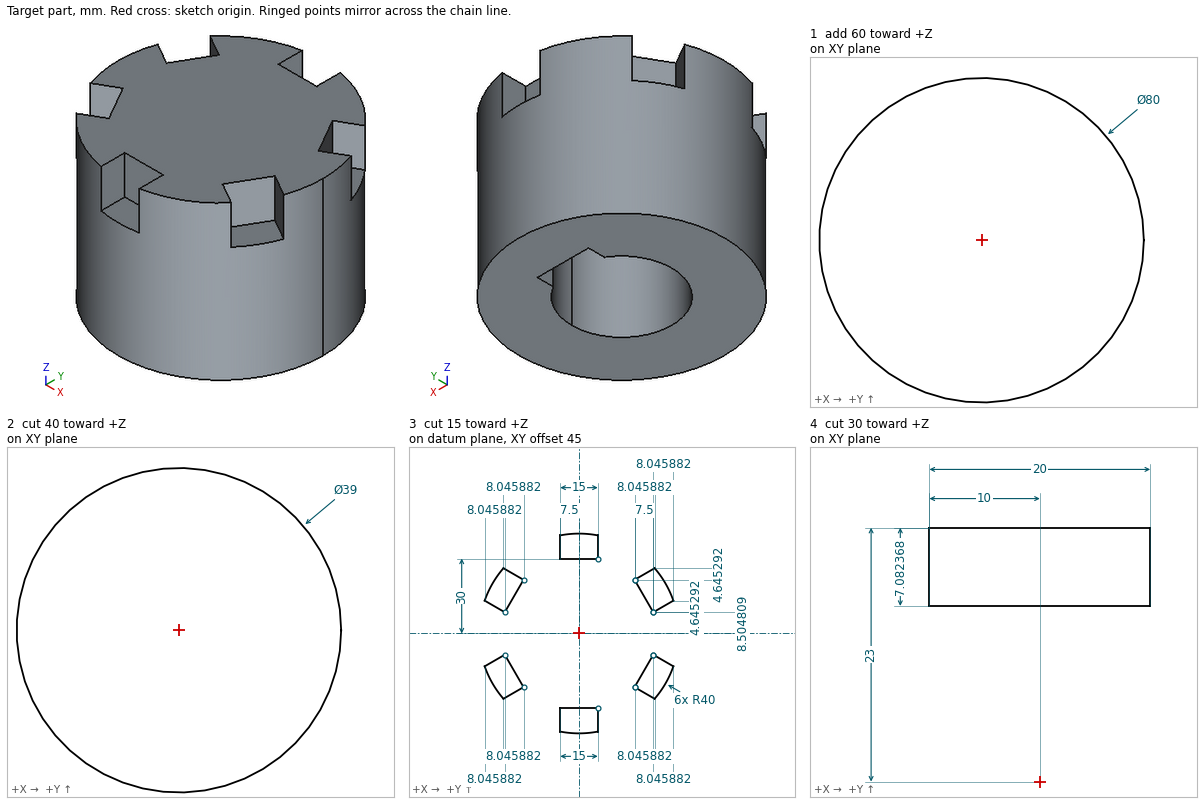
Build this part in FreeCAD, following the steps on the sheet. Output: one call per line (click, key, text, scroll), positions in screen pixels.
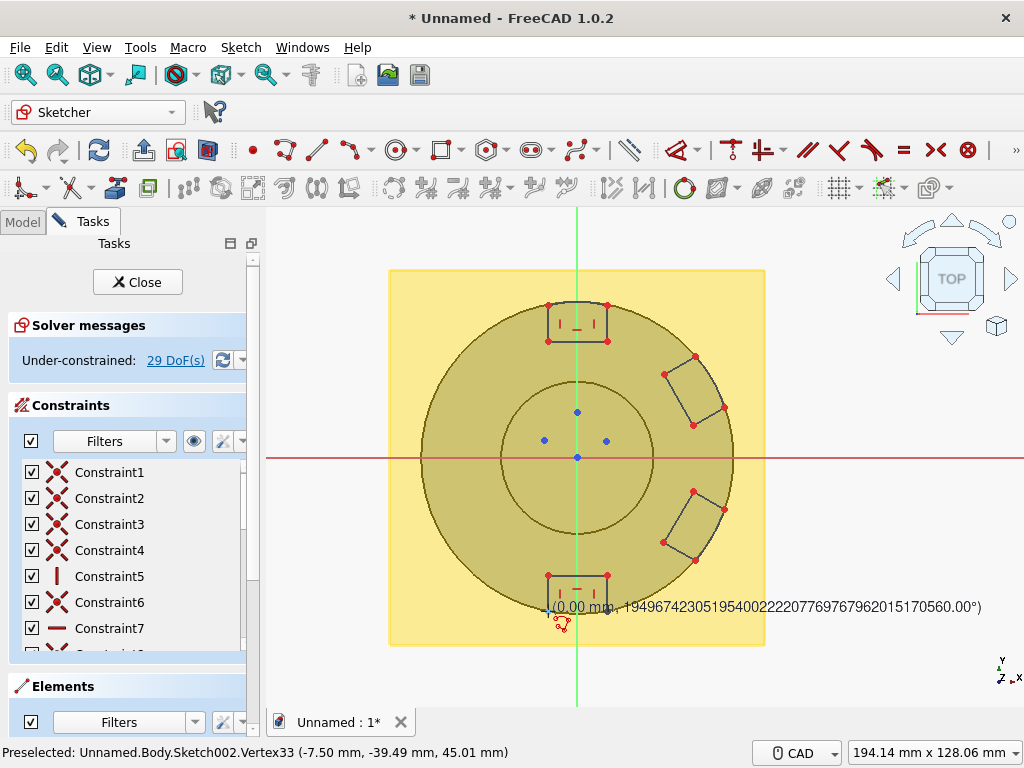
key(g)
key(3)
key(a)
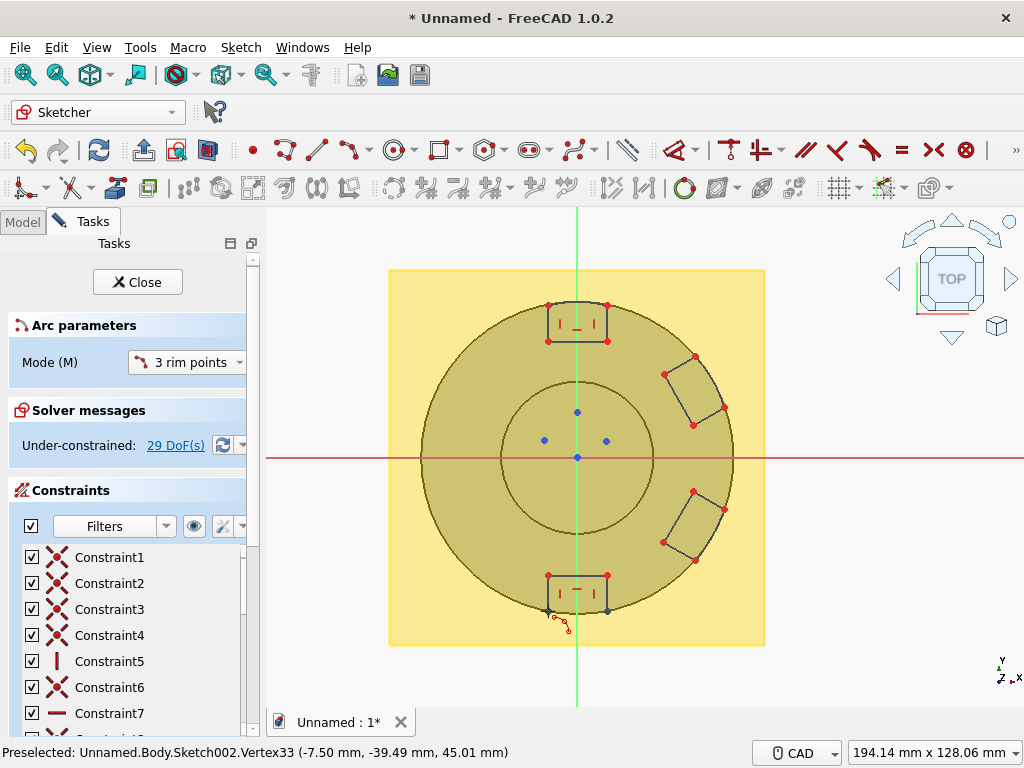
click(548, 612)
click(607, 612)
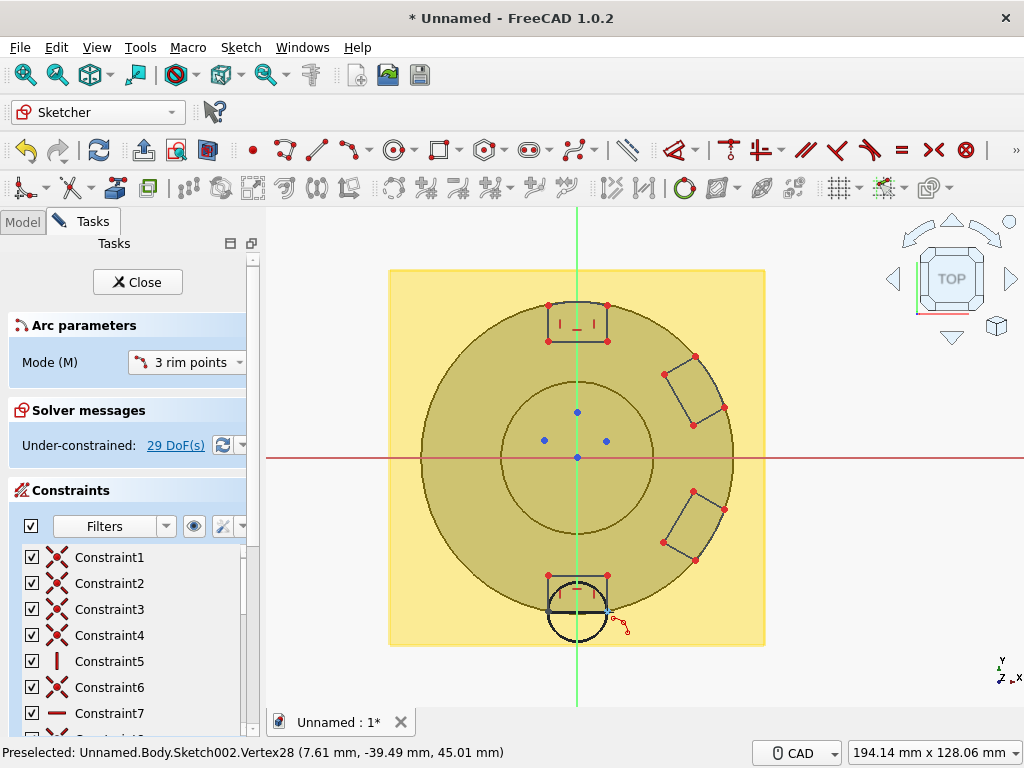
scroll(571, 614, up, 9)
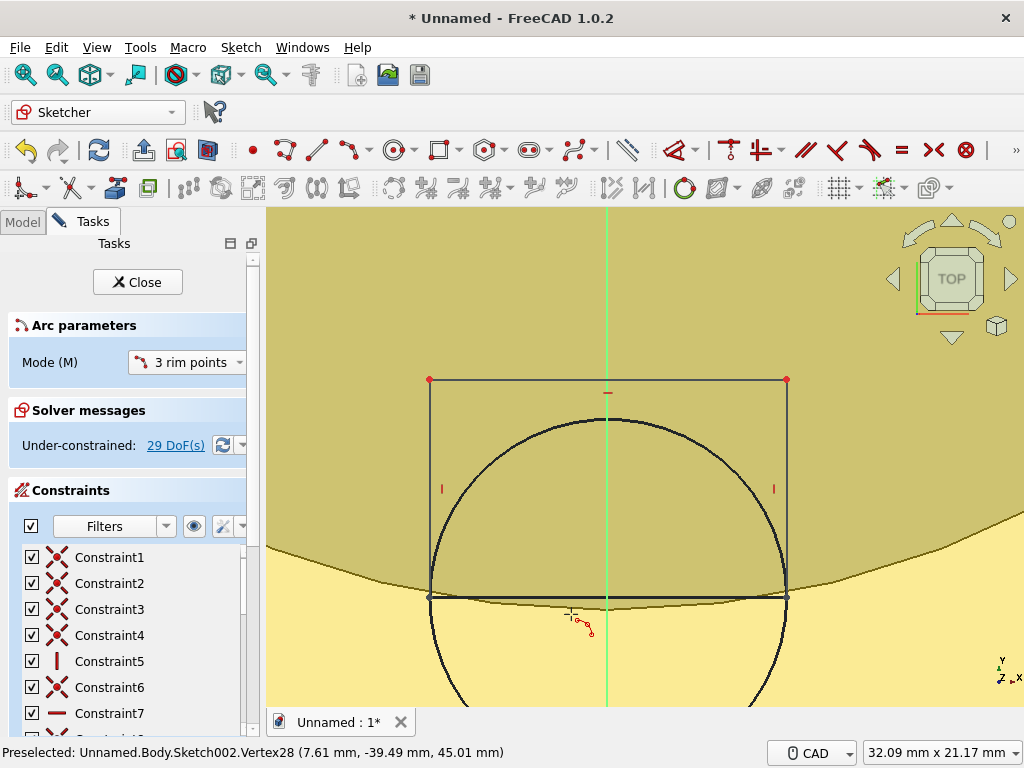
click(571, 609)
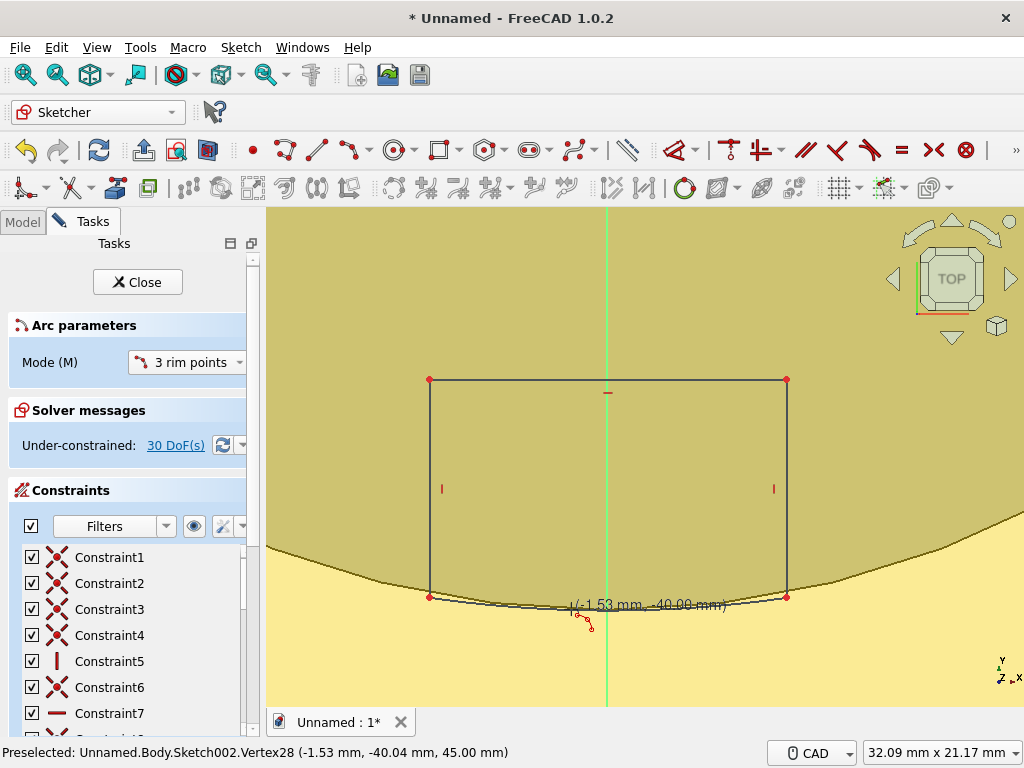
click(286, 150)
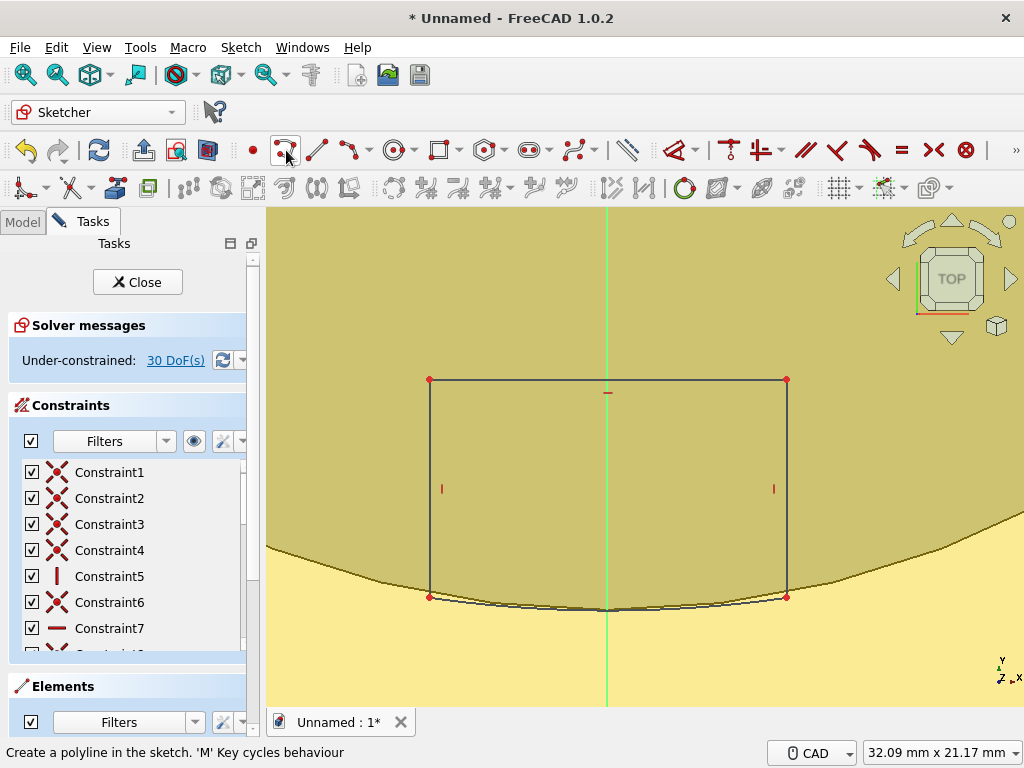
scroll(570, 614, down, 9)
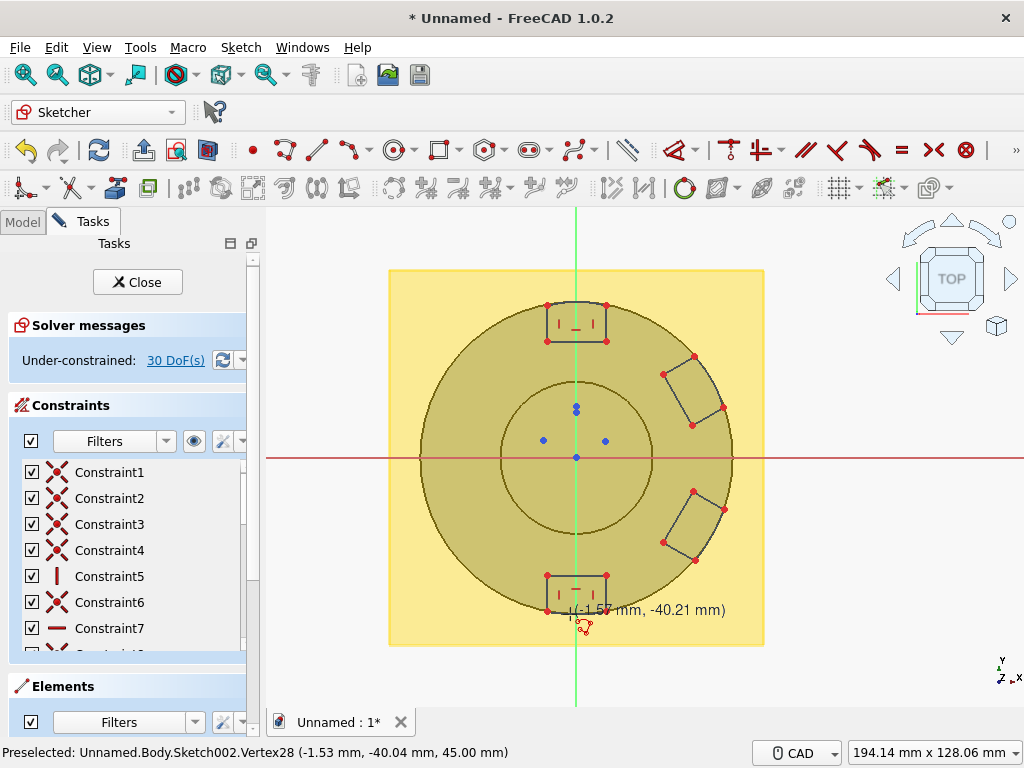
click(458, 560)
click(490, 542)
click(460, 491)
click(429, 509)
right_click(429, 509)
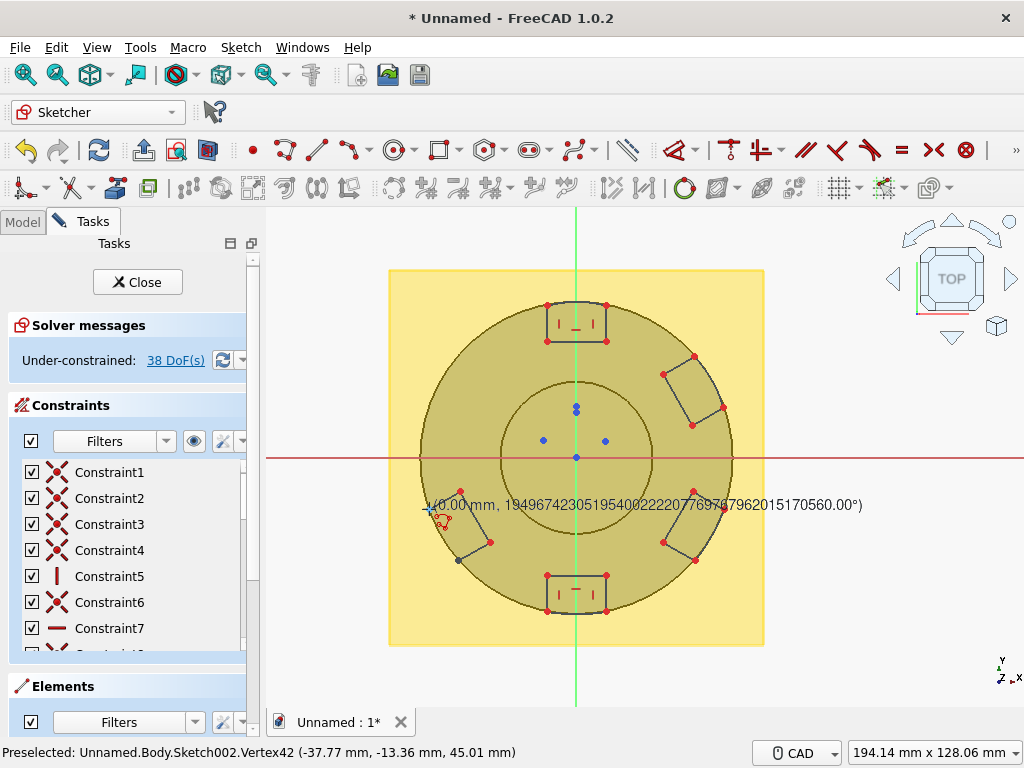
click(350, 150)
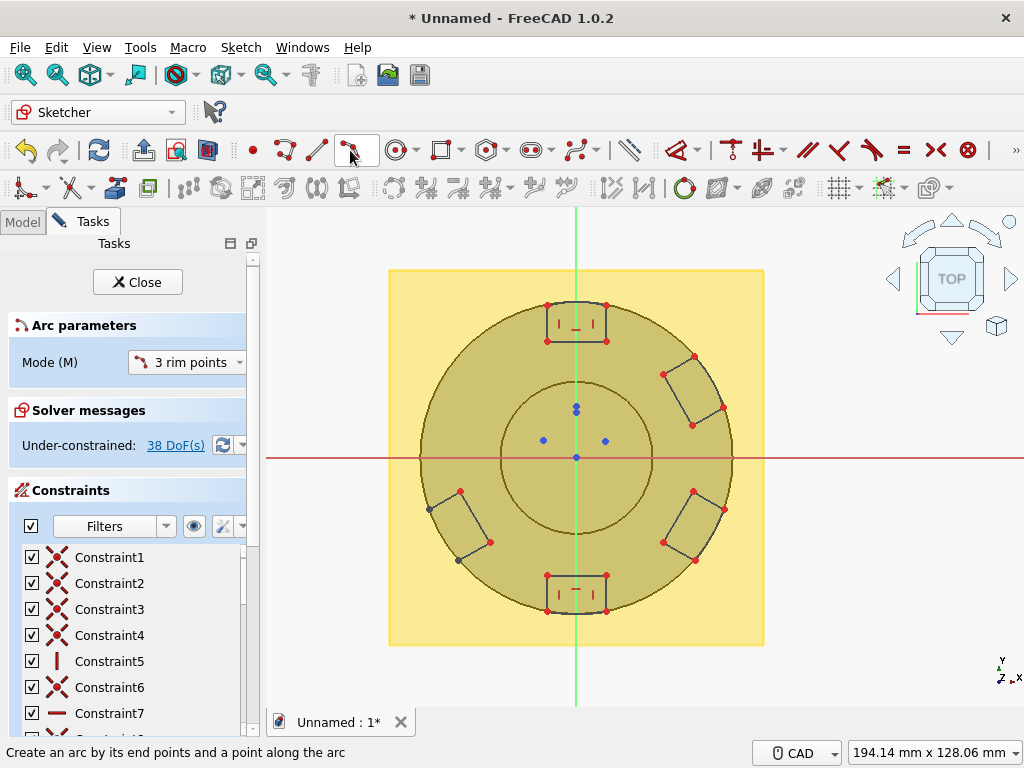
click(429, 510)
click(458, 561)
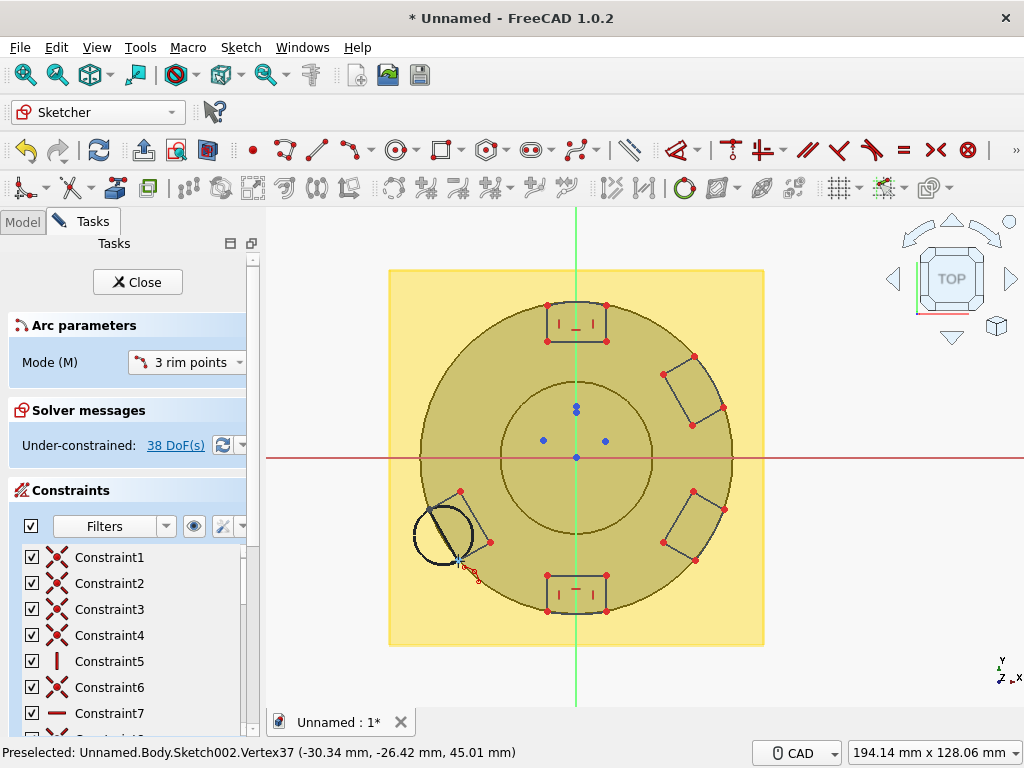
scroll(441, 536, up, 9)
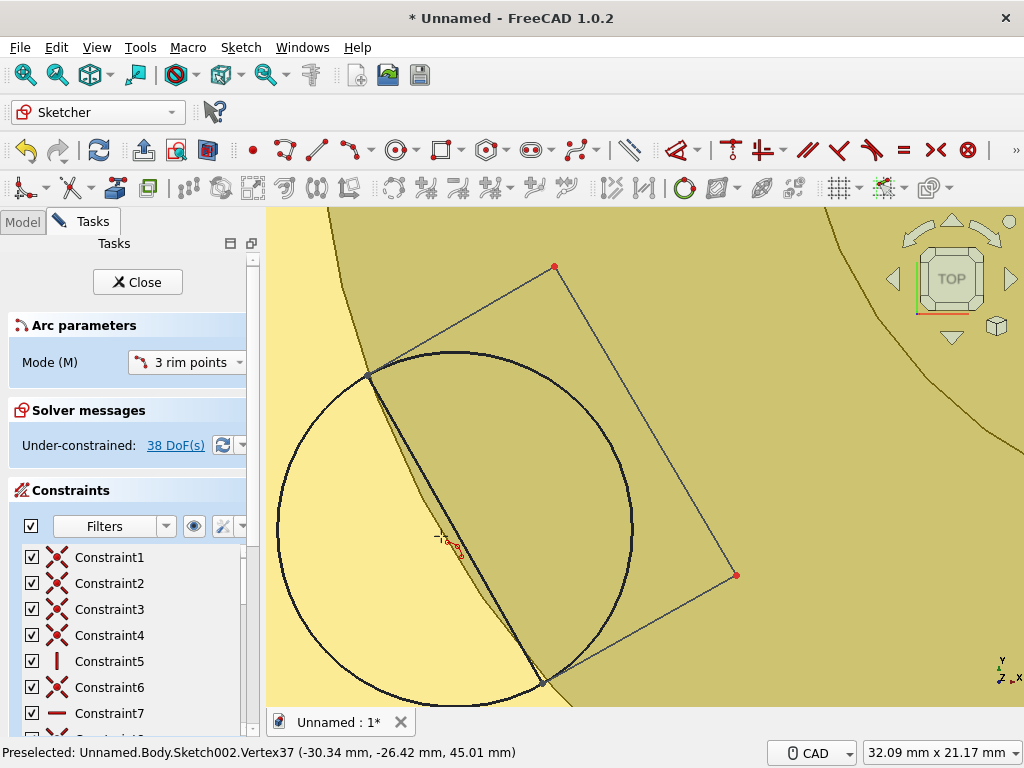
click(441, 532)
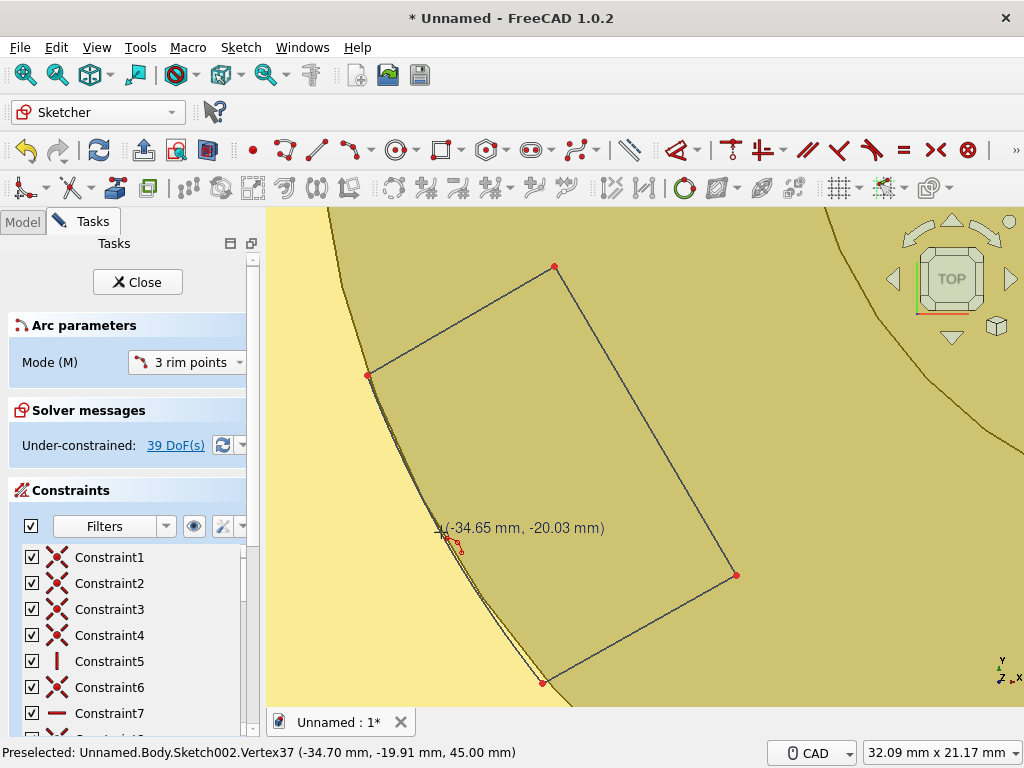
click(286, 150)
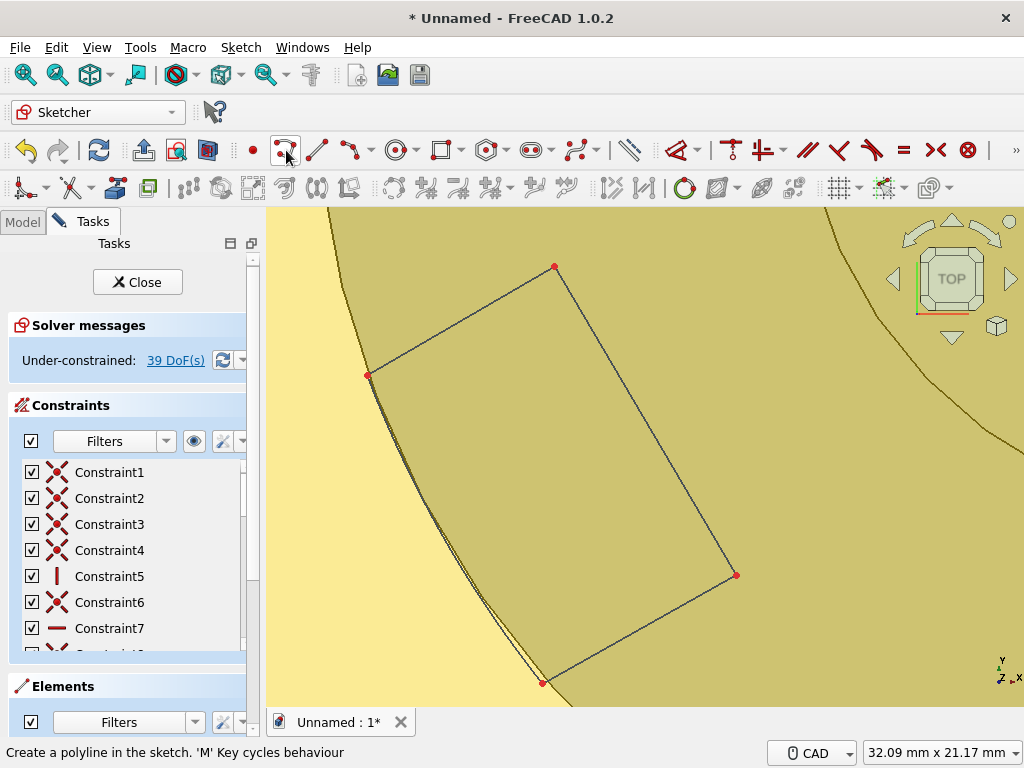
scroll(441, 536, down, 9)